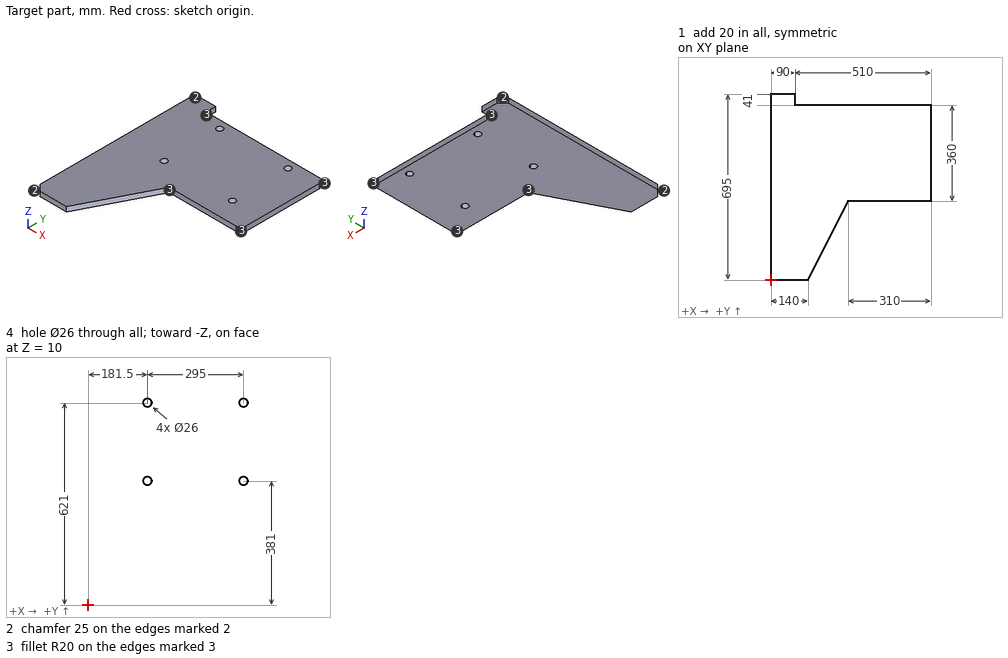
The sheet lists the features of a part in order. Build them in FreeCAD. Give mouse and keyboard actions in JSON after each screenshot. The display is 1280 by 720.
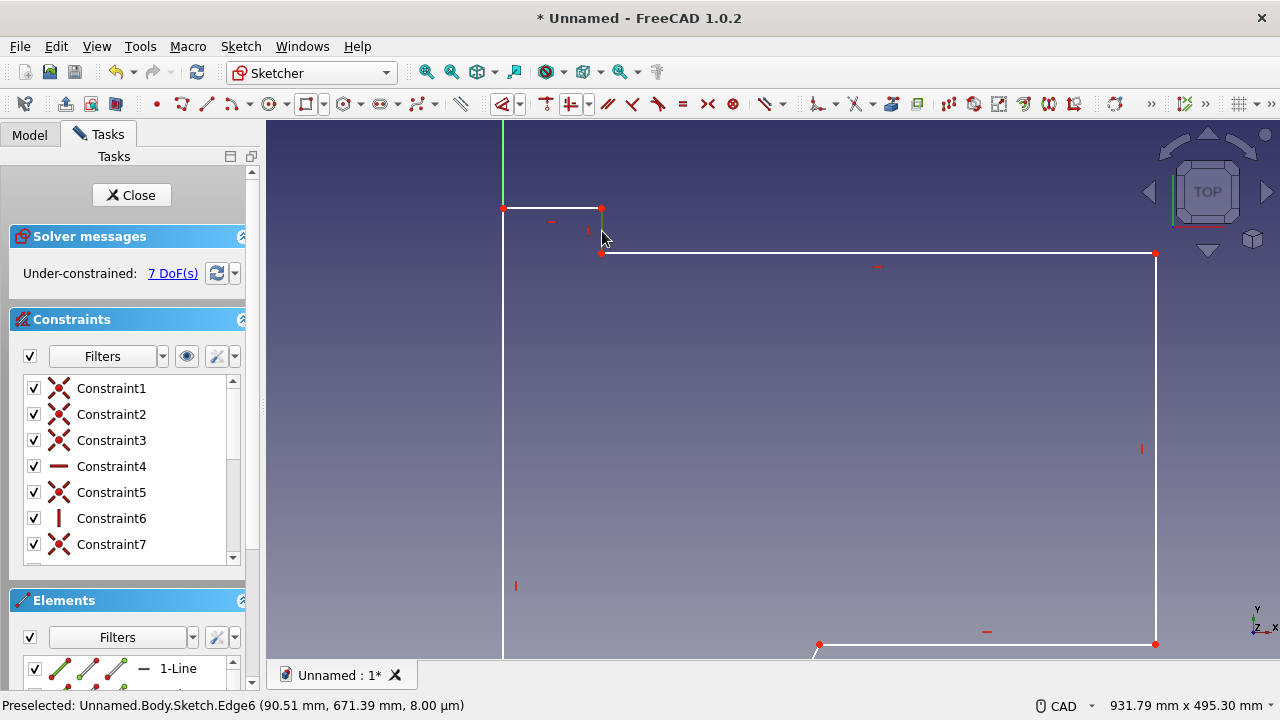
{"action": "left_click", "coordinate": [520, 104]}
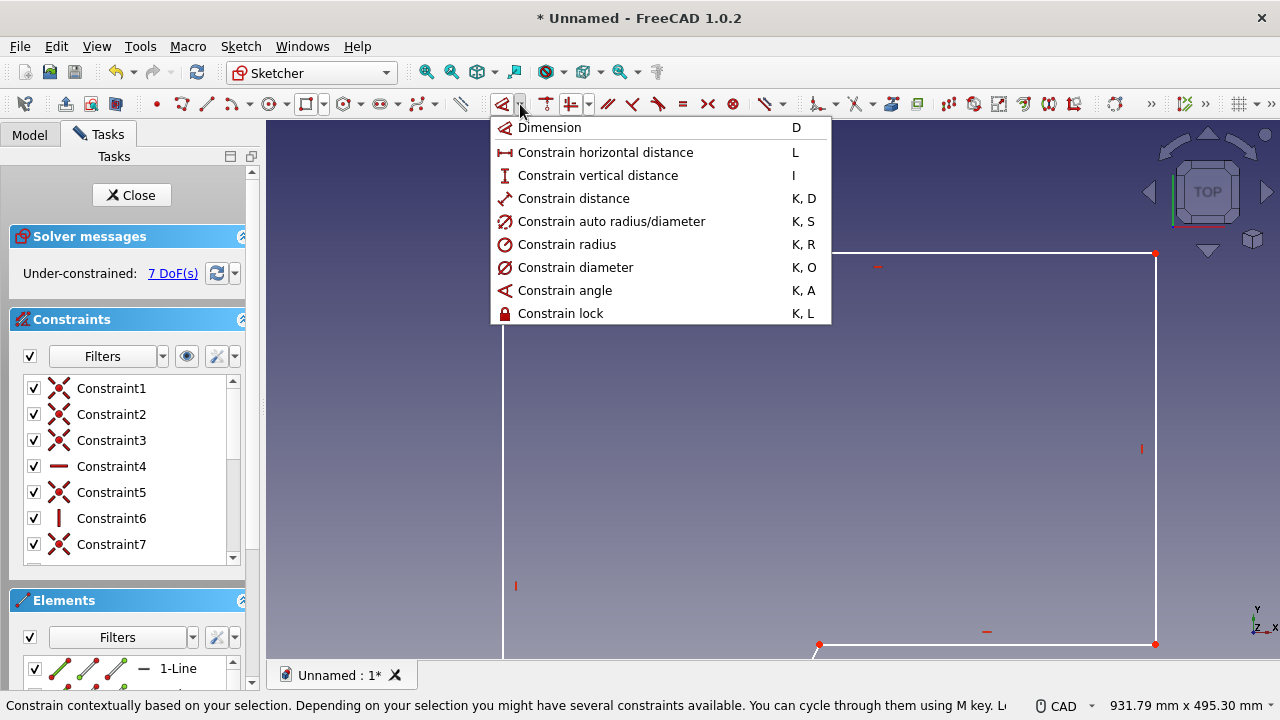
{"action": "left_click", "coordinate": [661, 176]}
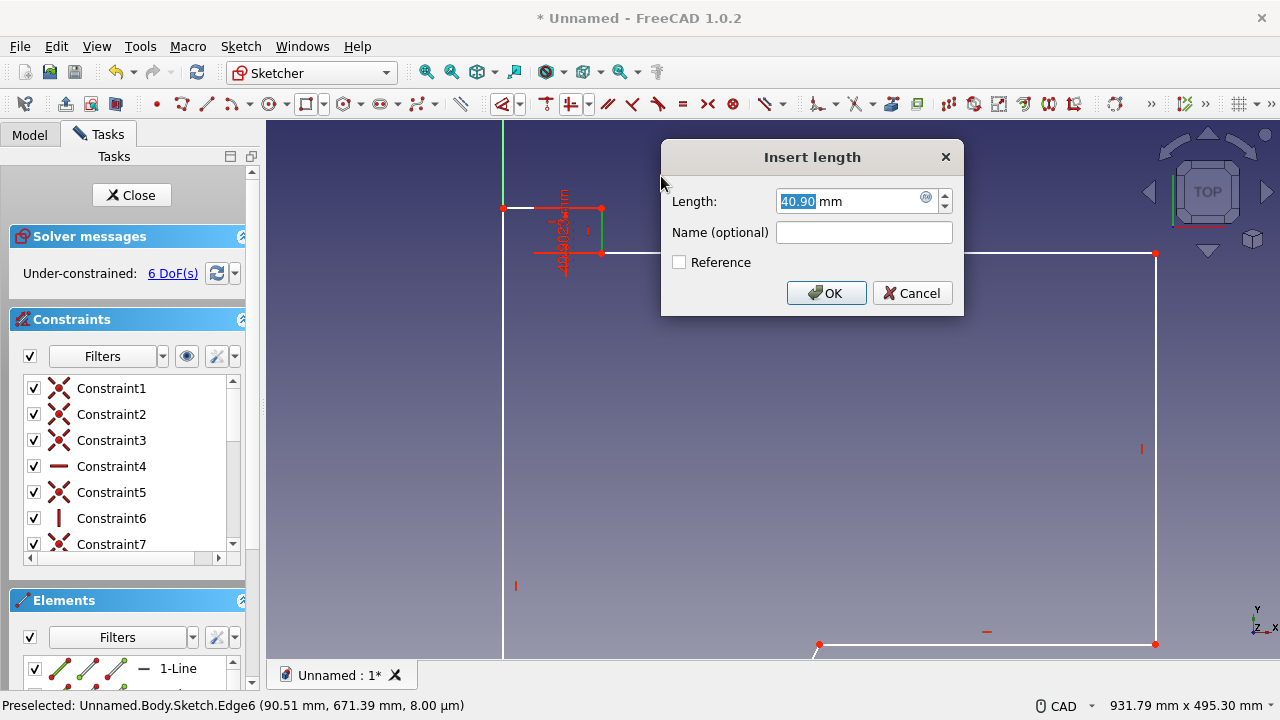
{"action": "type", "text": "41"}
{"action": "key", "text": "Return"}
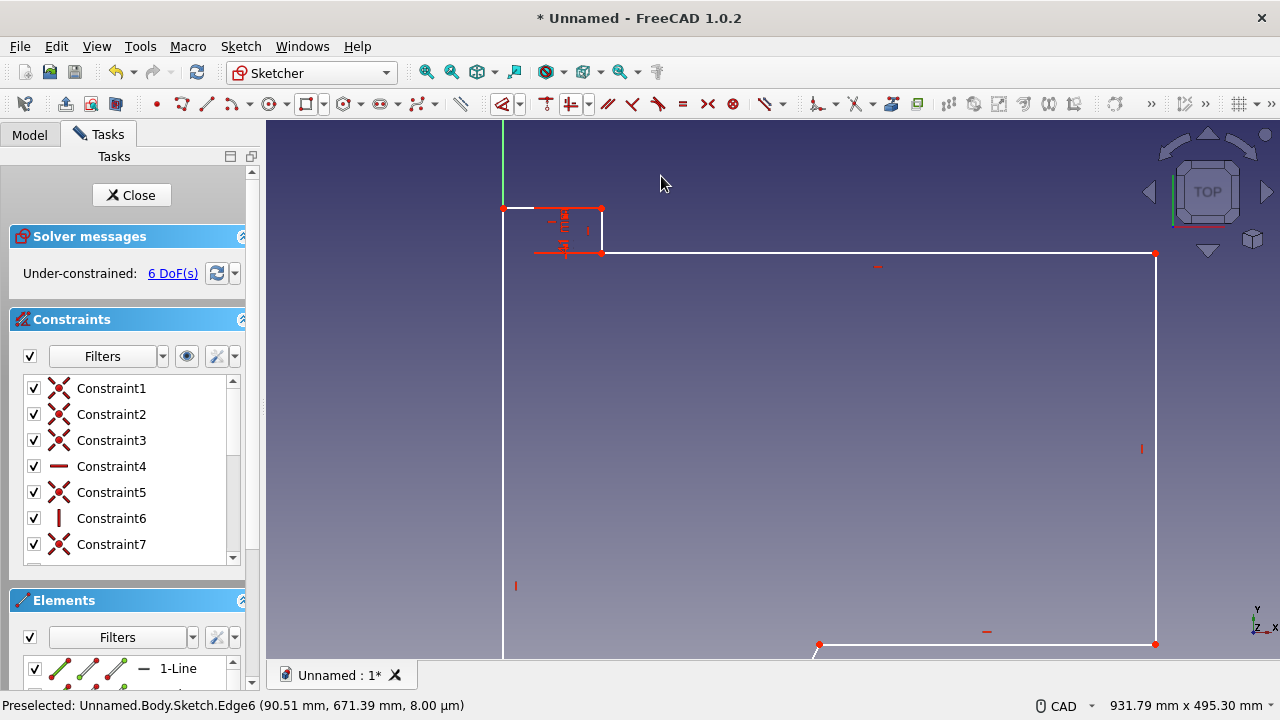
{"action": "left_click", "coordinate": [533, 208]}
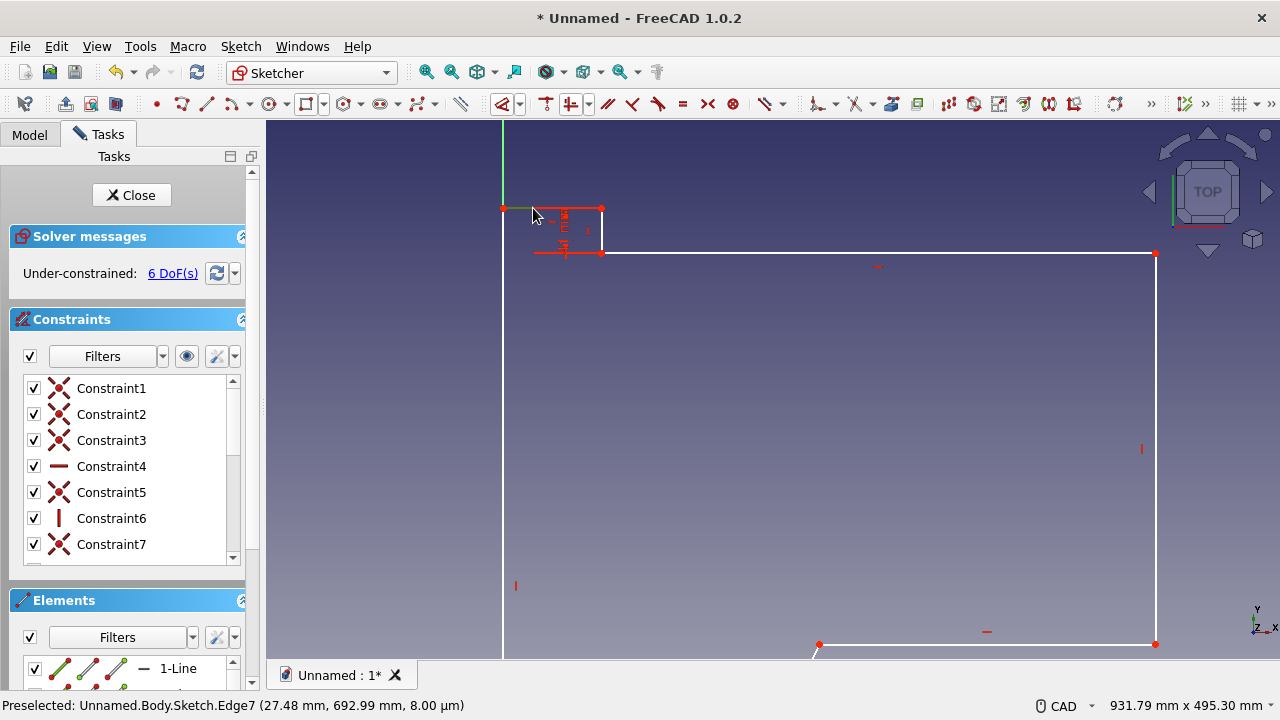
{"action": "key", "text": "l"}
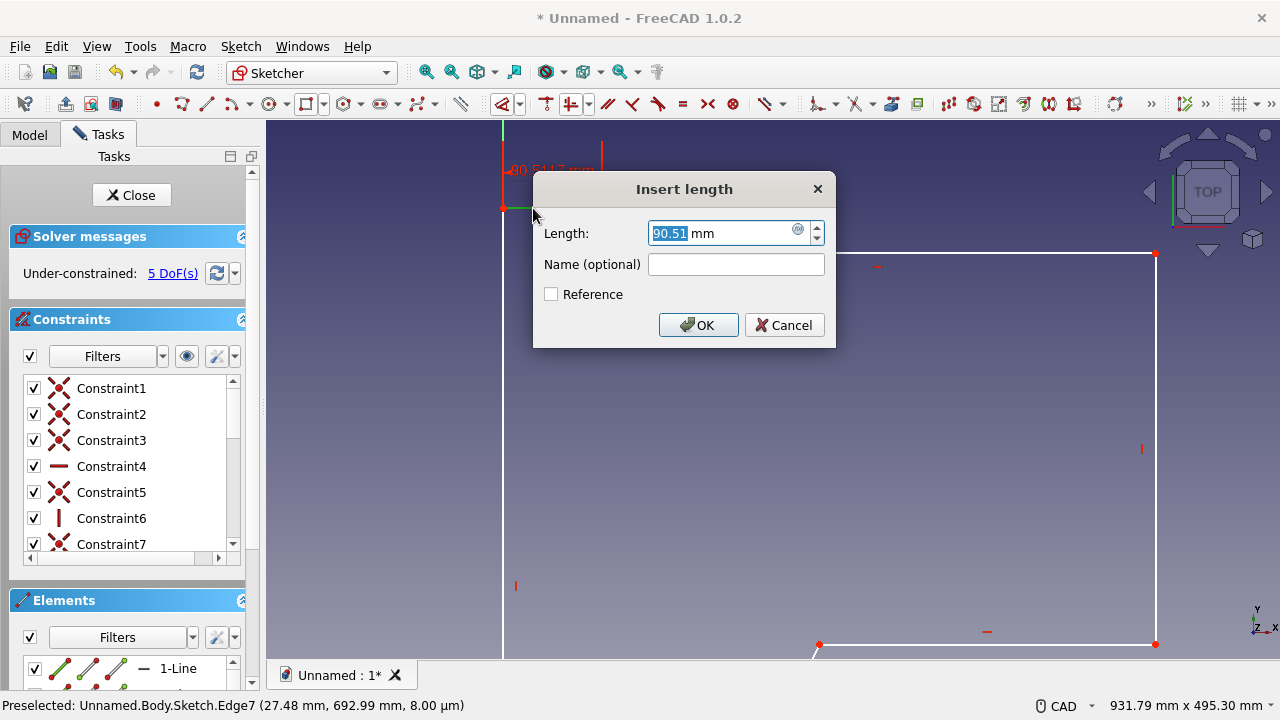
{"action": "type", "text": "90"}
{"action": "key", "text": "Return"}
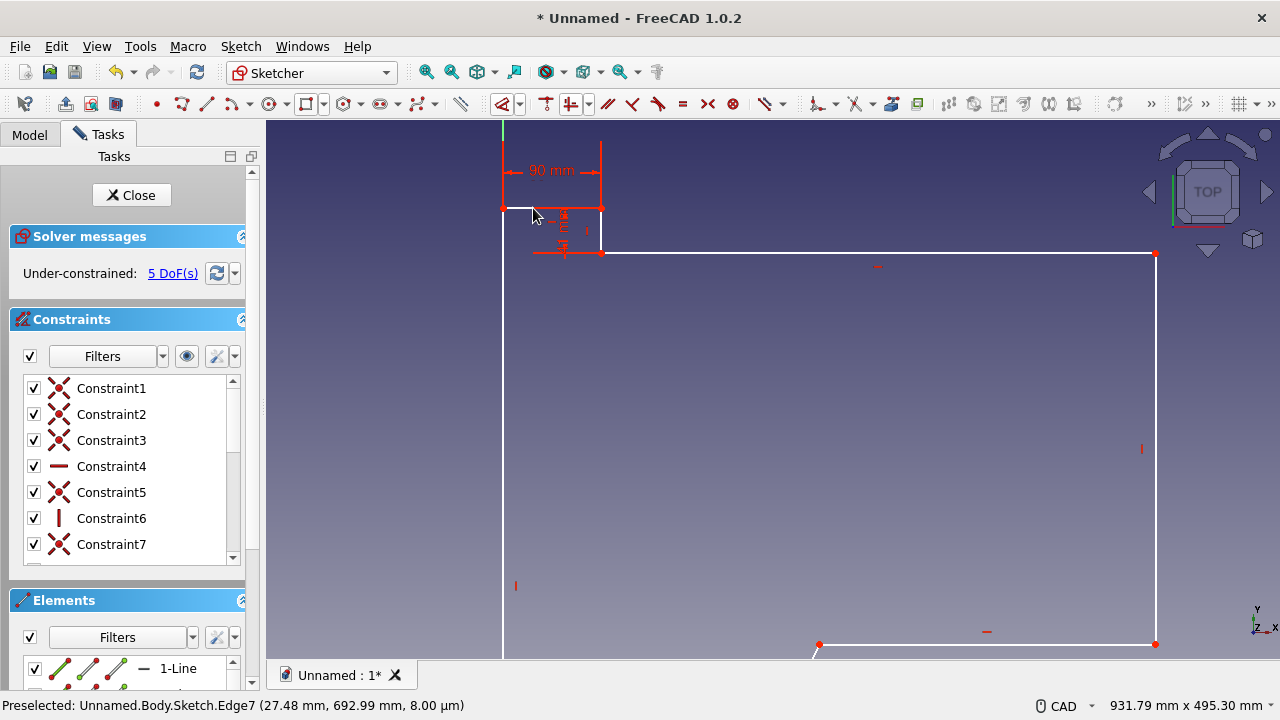
{"action": "scroll", "coordinate": [602, 230], "scroll_direction": "down", "scroll_amount": 4}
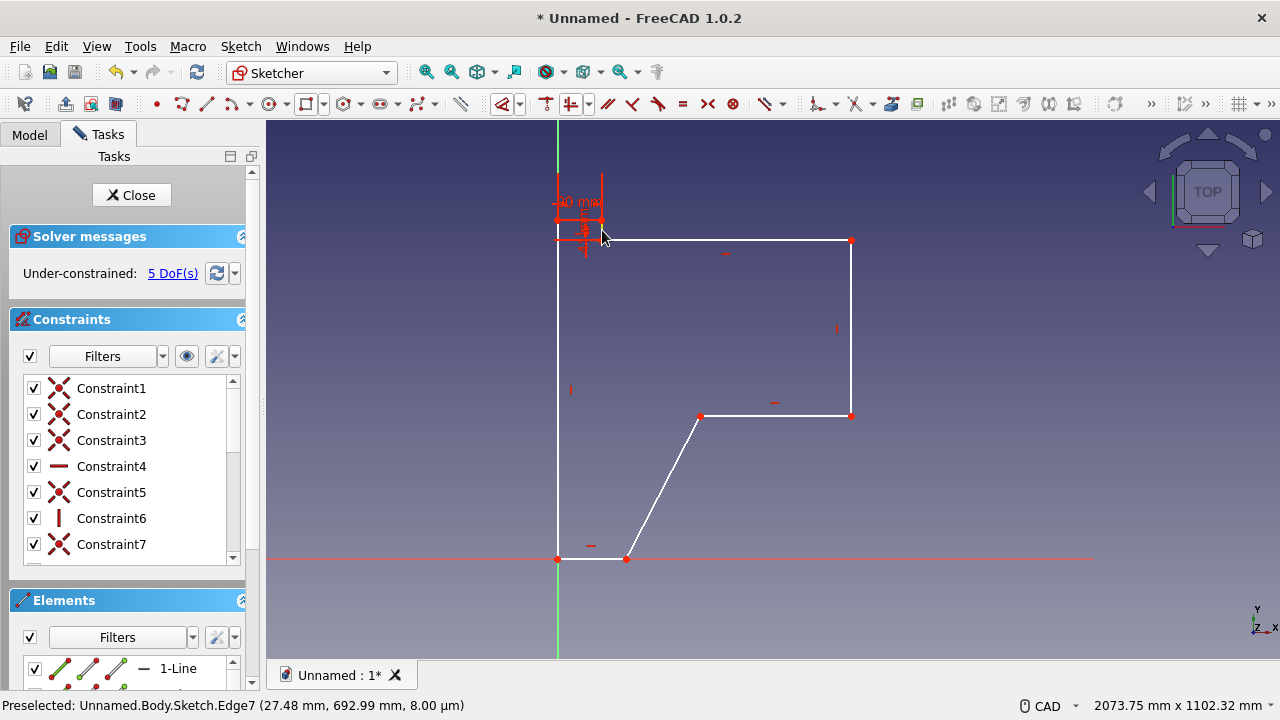
{"action": "left_click", "coordinate": [578, 559]}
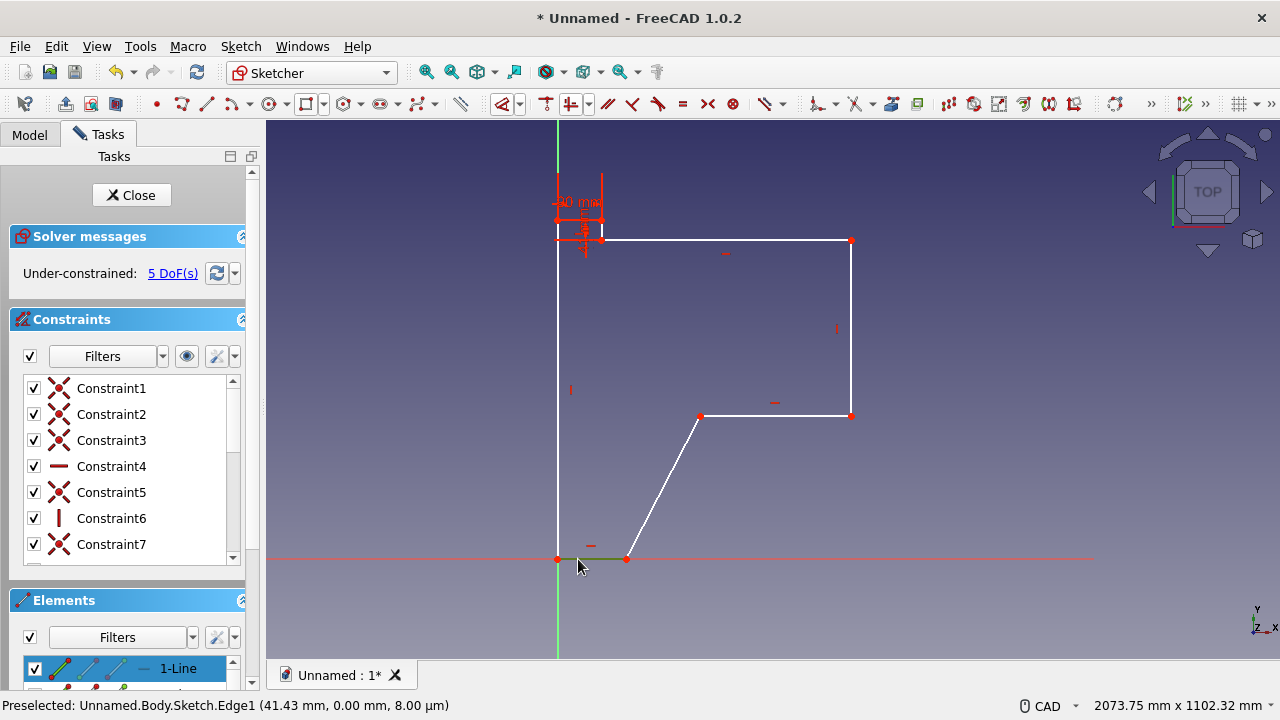
{"action": "key", "text": "l"}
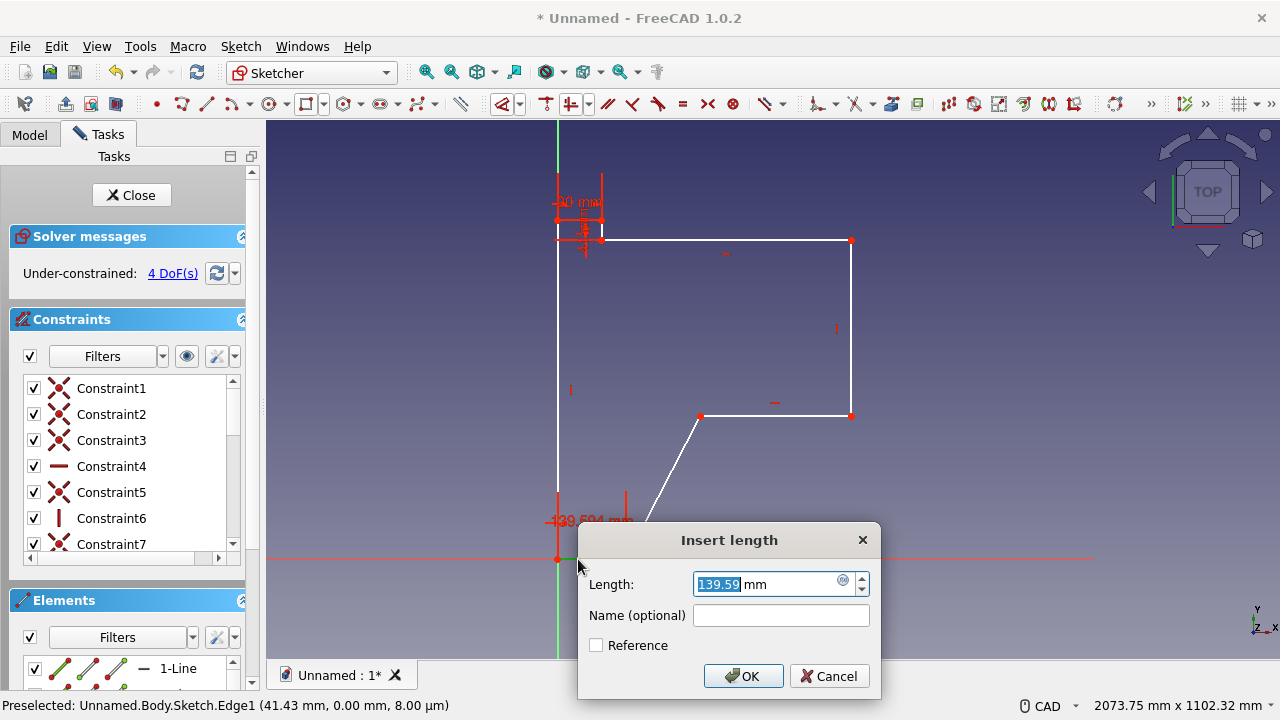
{"action": "type", "text": "140"}
{"action": "key", "text": "Return"}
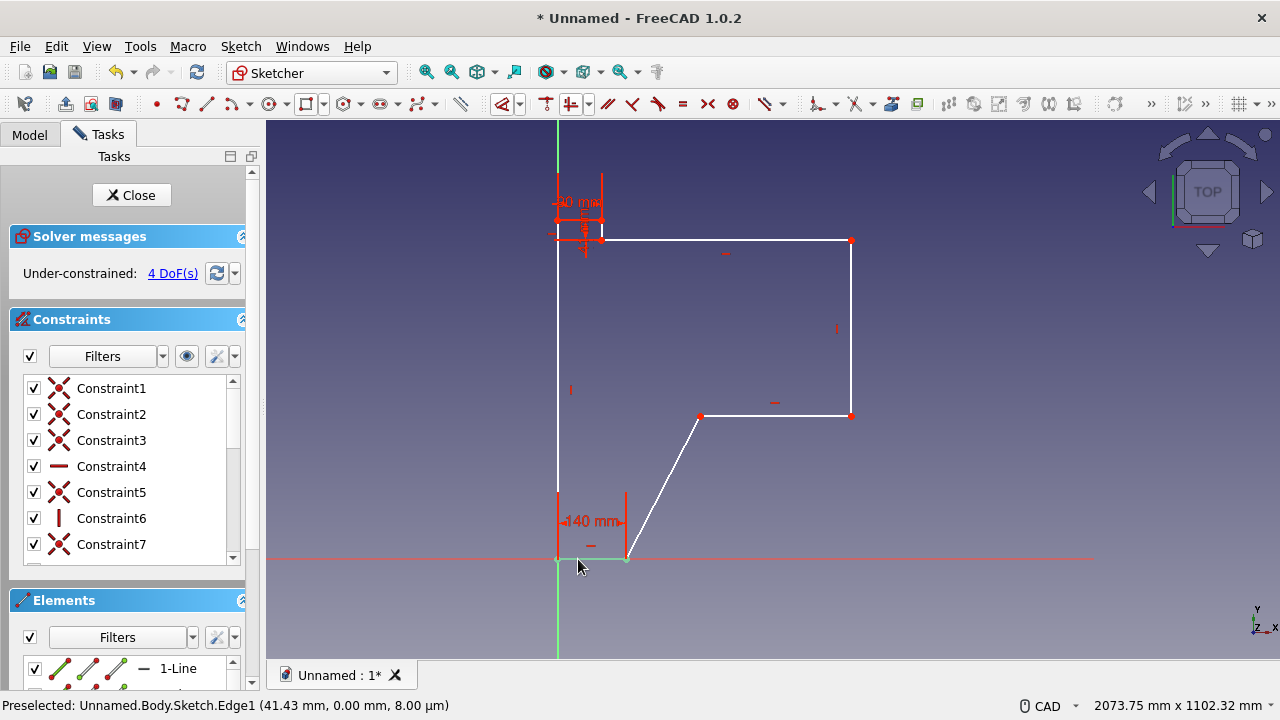
{"action": "left_click", "coordinate": [745, 416]}